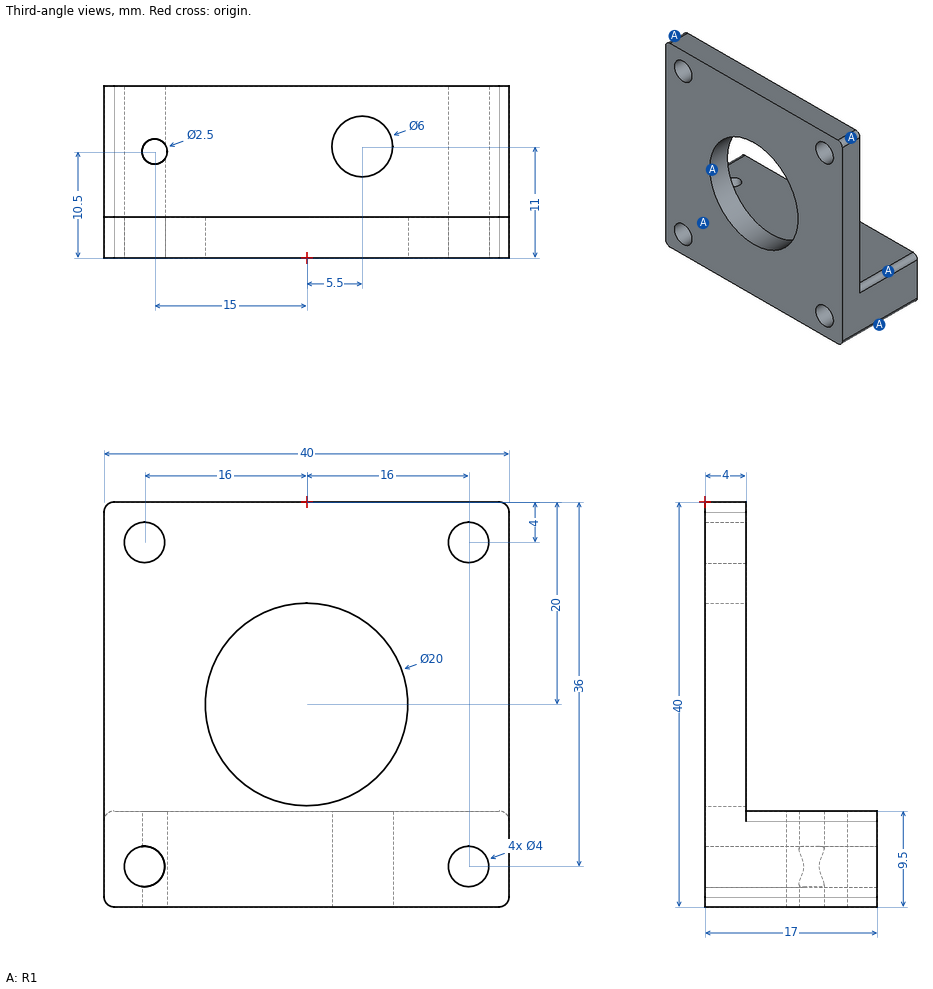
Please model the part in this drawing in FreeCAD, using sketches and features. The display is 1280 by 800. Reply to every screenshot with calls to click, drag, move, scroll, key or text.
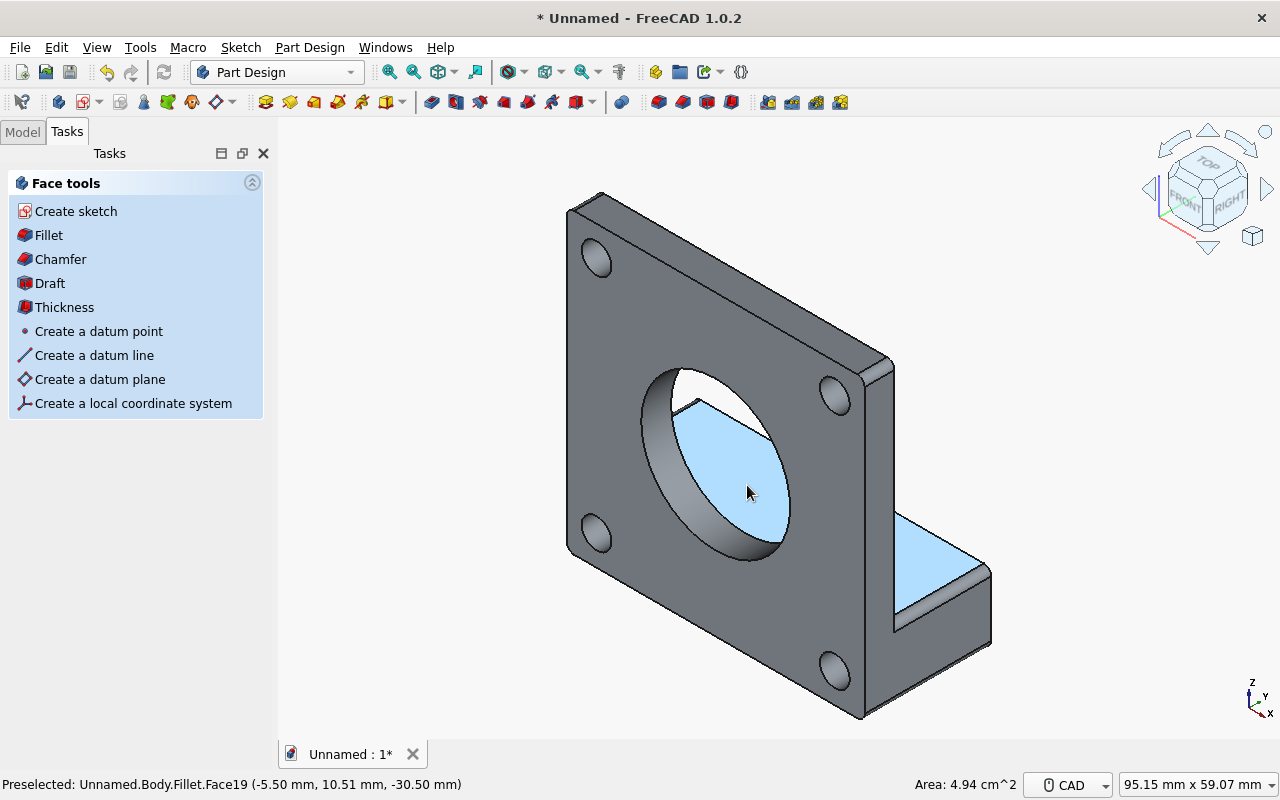
click(84, 102)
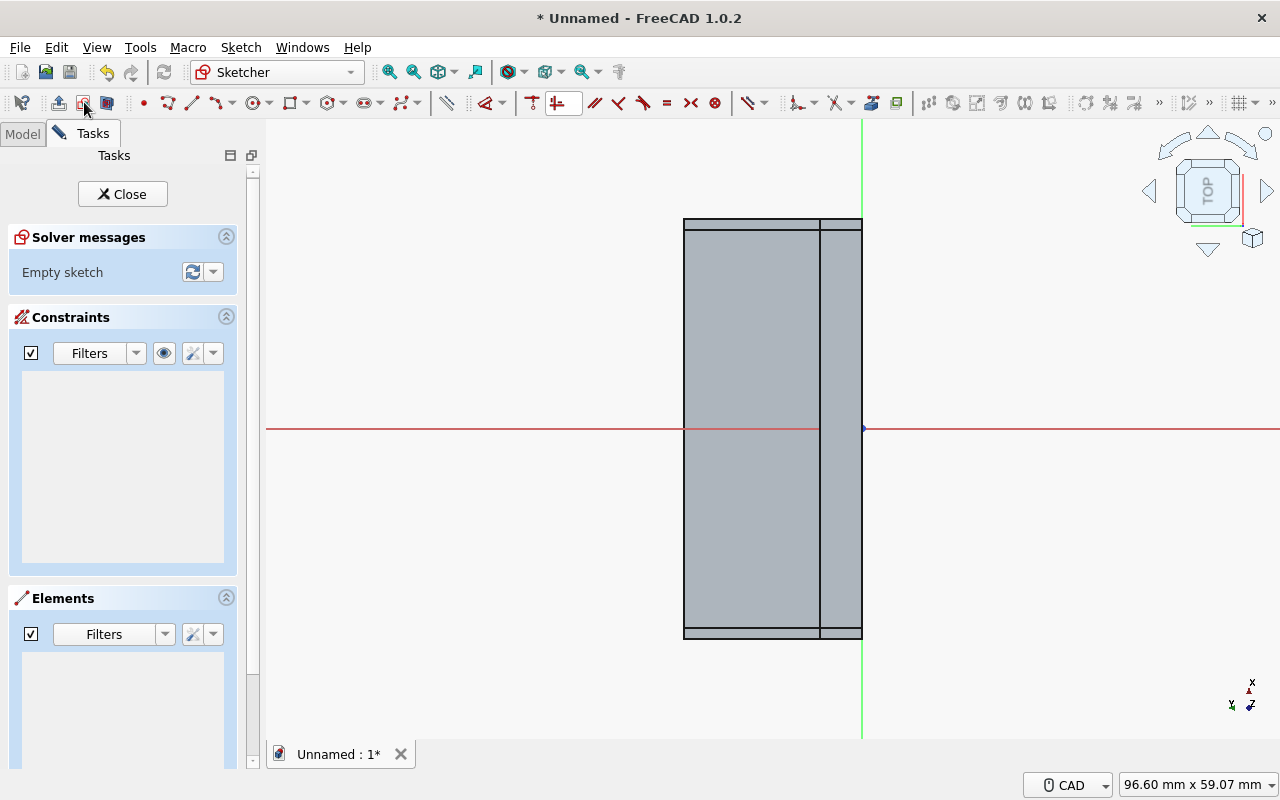
scroll(960, 552, up, 2)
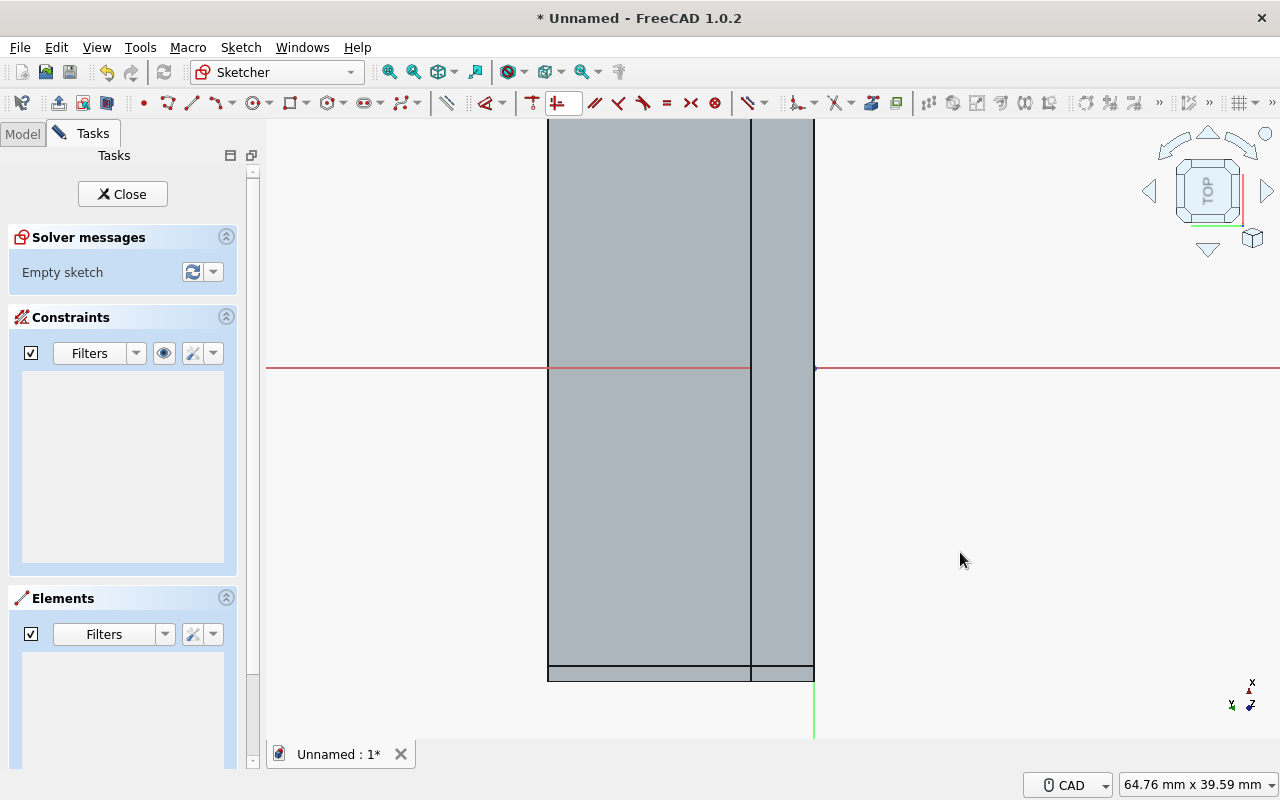
click(254, 104)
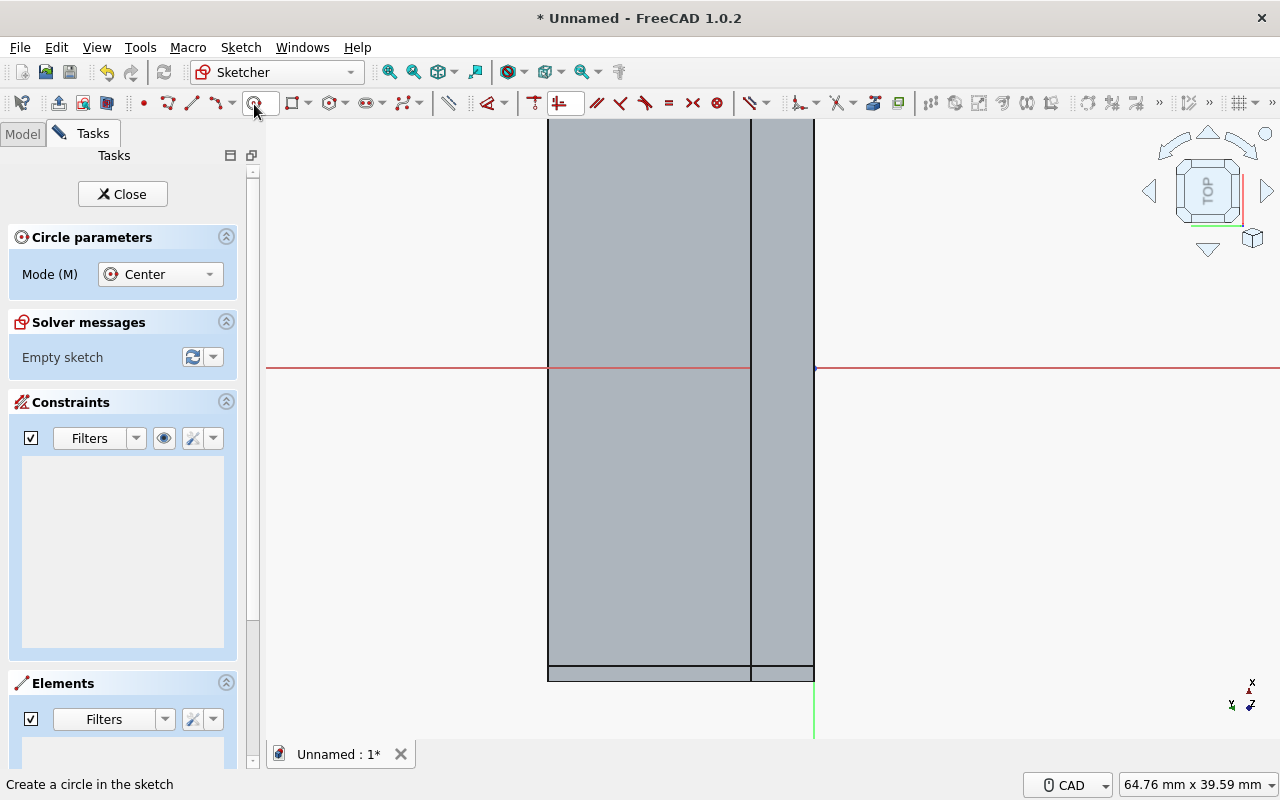
click(642, 282)
move(675, 249)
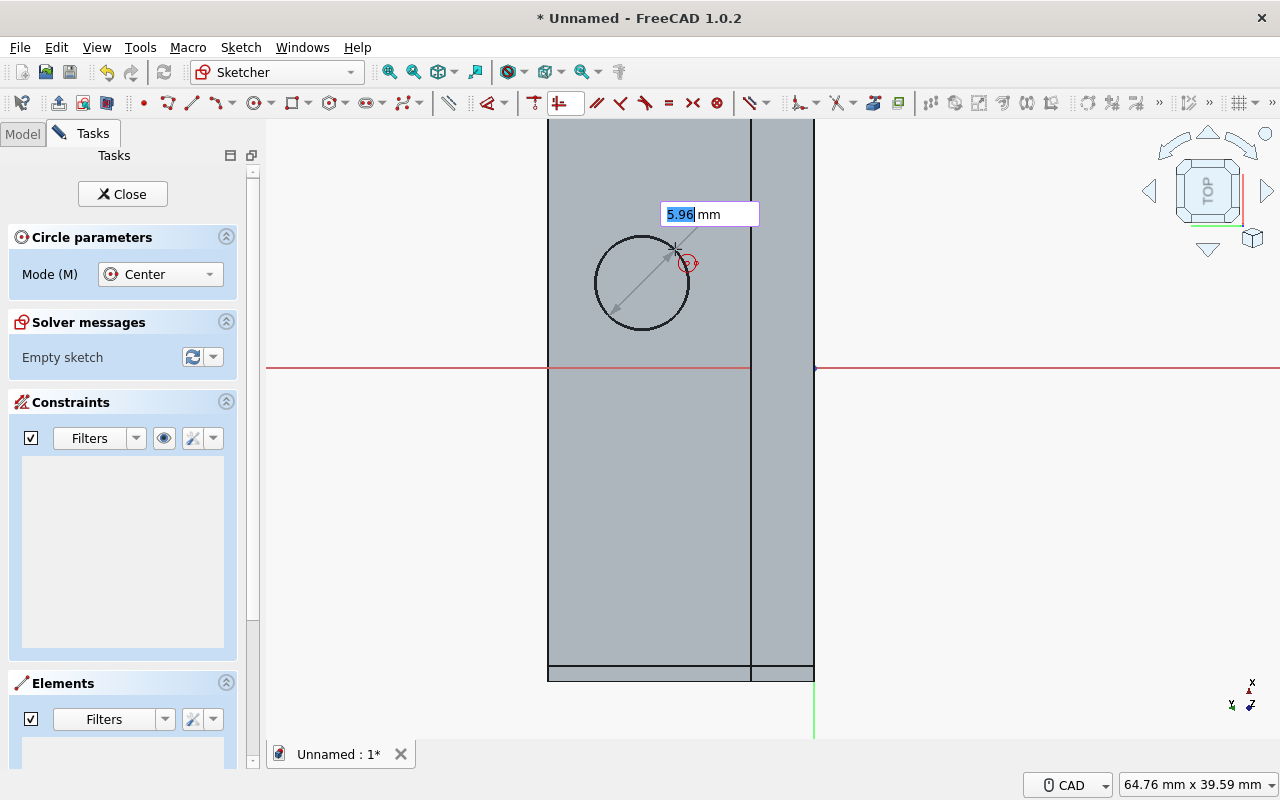
text(6)
key(Return)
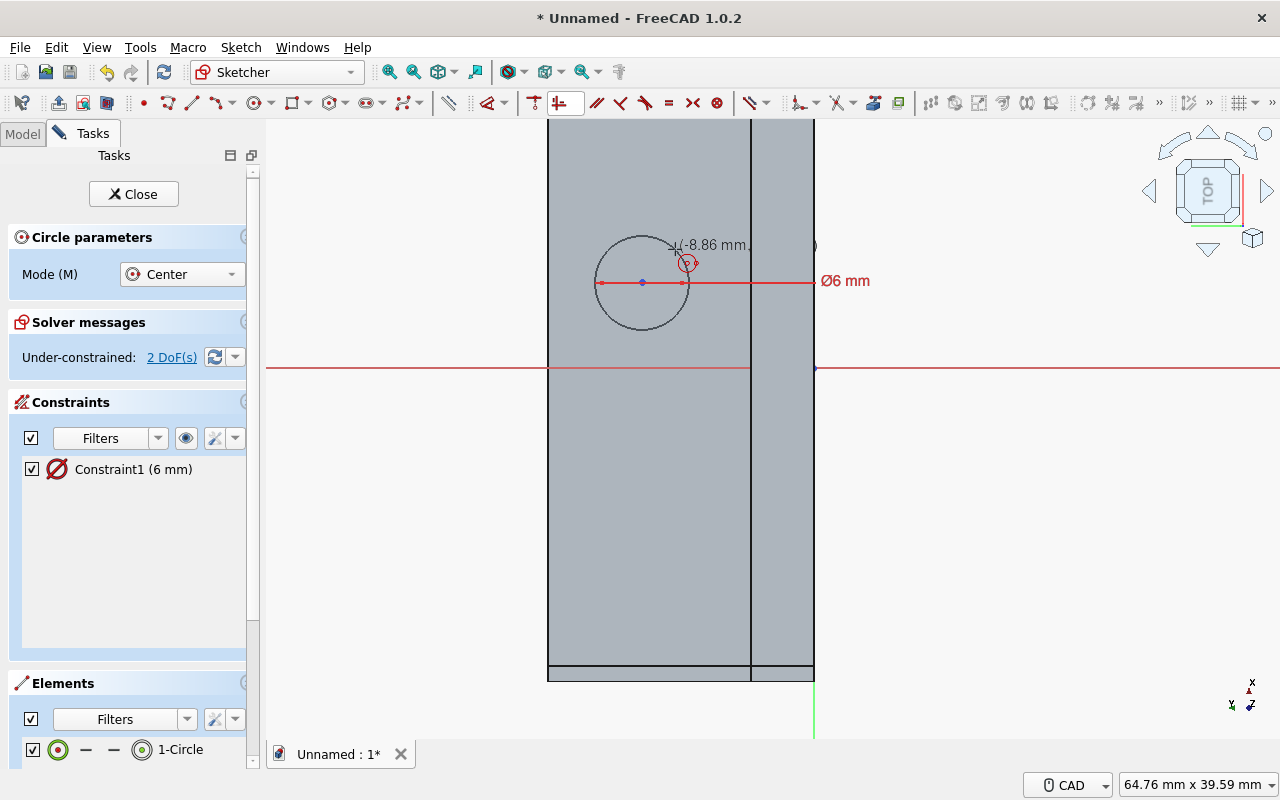
click(649, 603)
move(663, 589)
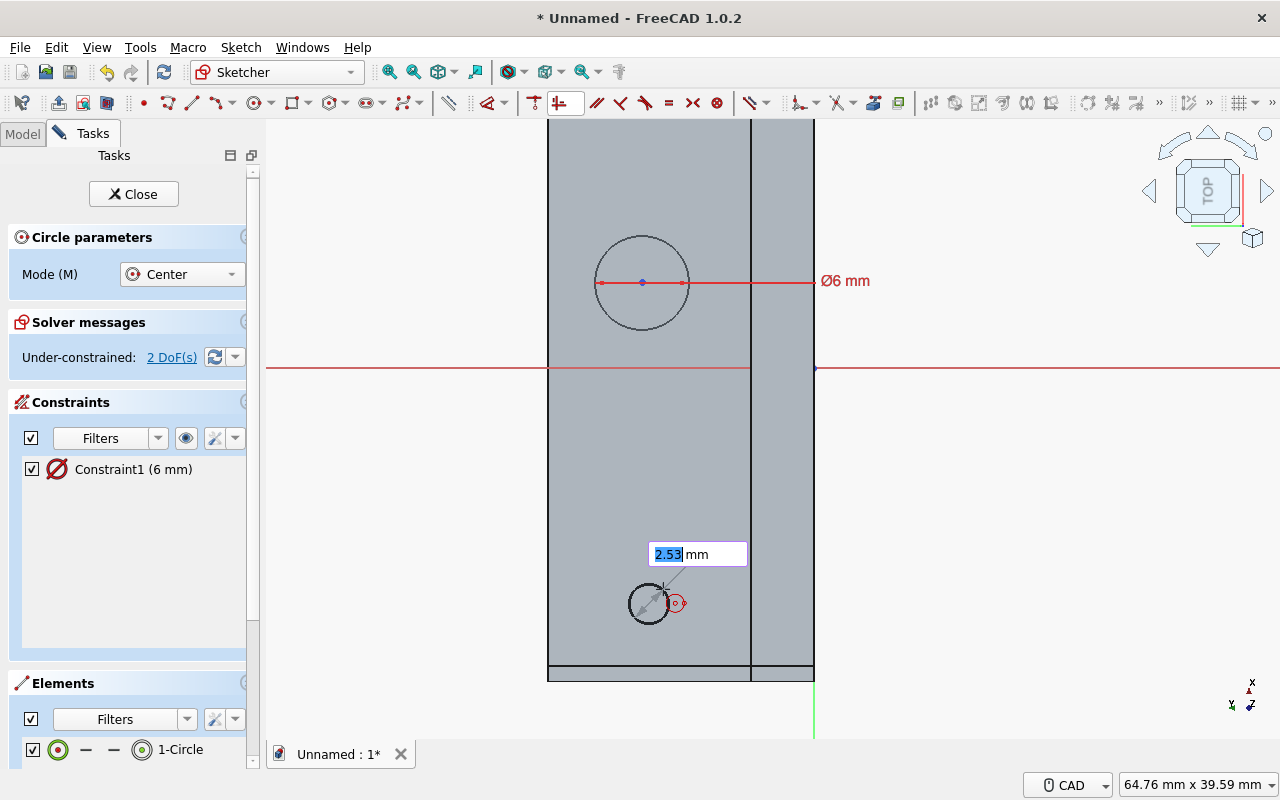
text(2.5)
key(Return)
key(Escape)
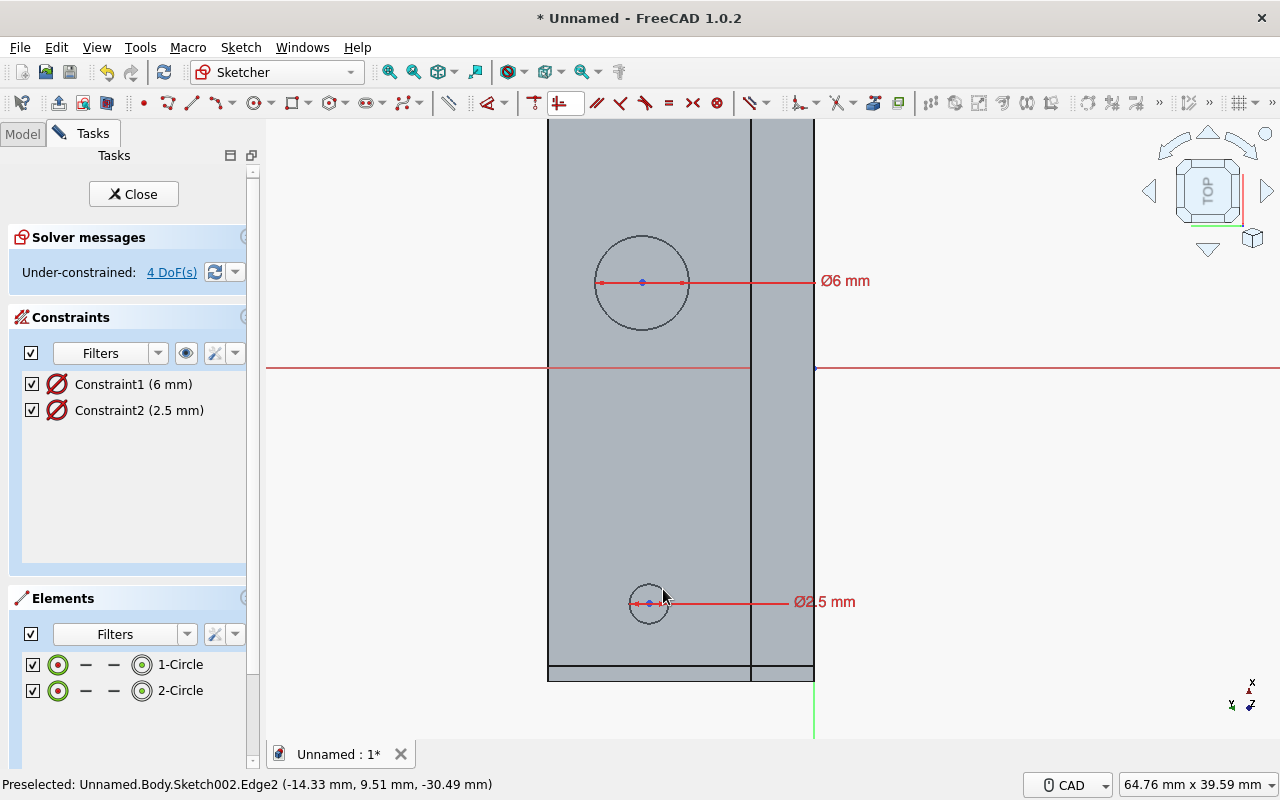
click(488, 104)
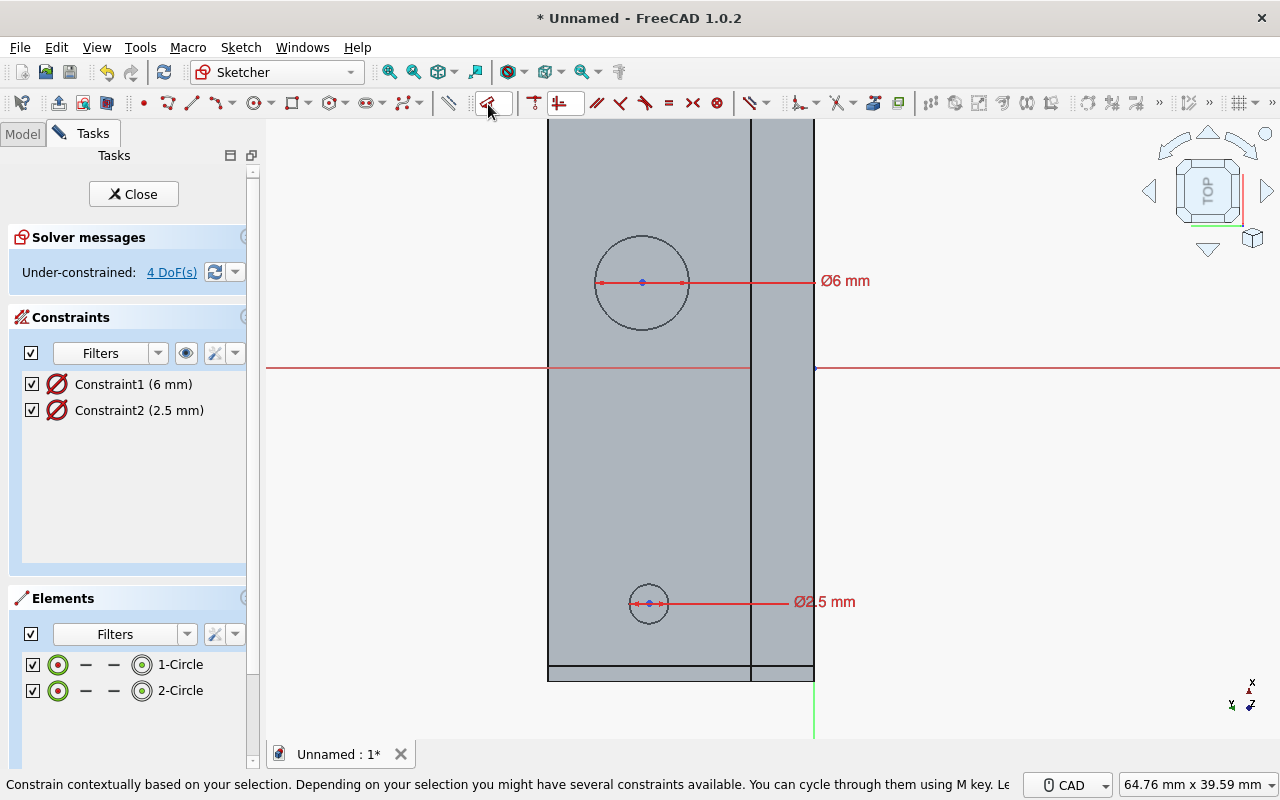
click(642, 283)
click(728, 249)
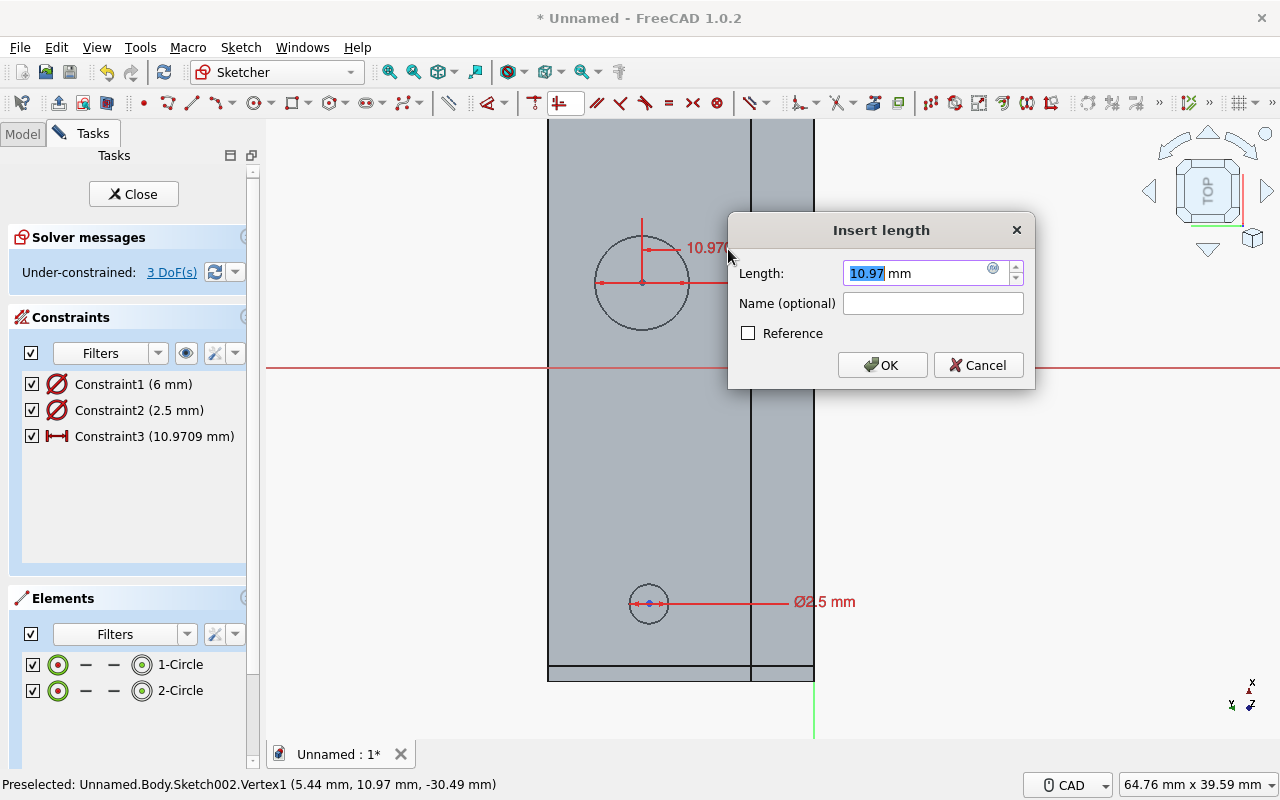
text(11)
key(Return)